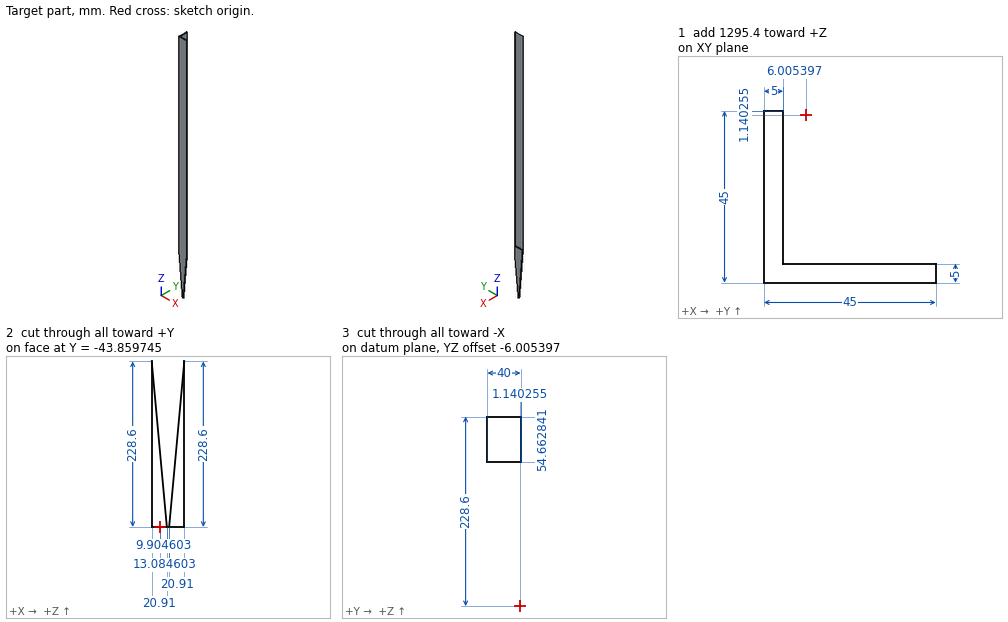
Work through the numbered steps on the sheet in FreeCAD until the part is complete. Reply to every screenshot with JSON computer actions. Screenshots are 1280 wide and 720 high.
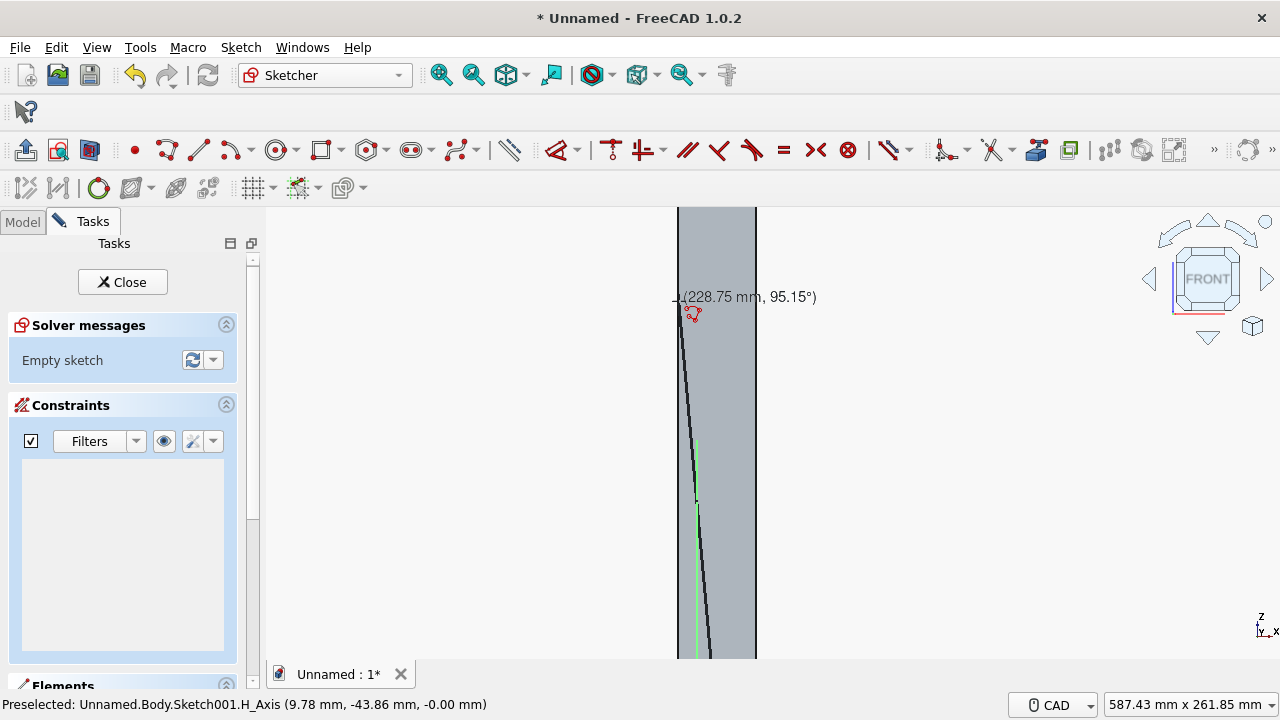
{"action": "left_click", "coordinate": [678, 301]}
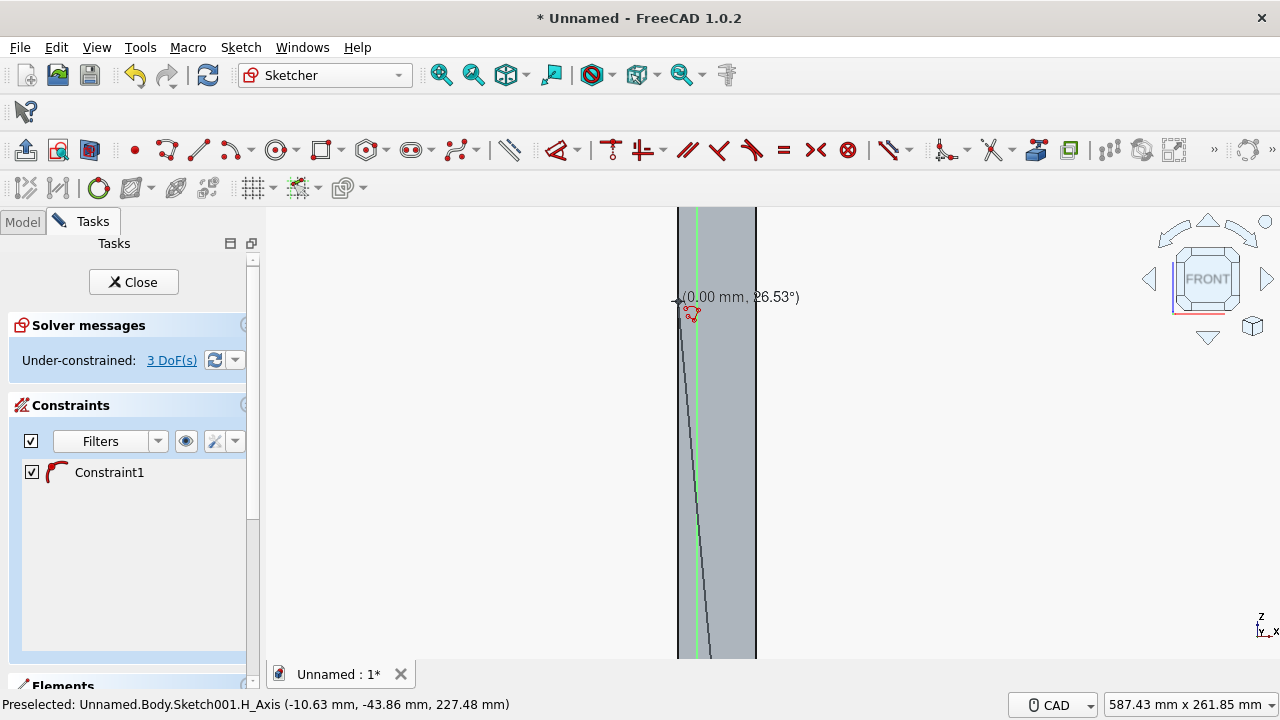
{"action": "scroll", "coordinate": [679, 300], "scroll_direction": "down", "scroll_amount": 2}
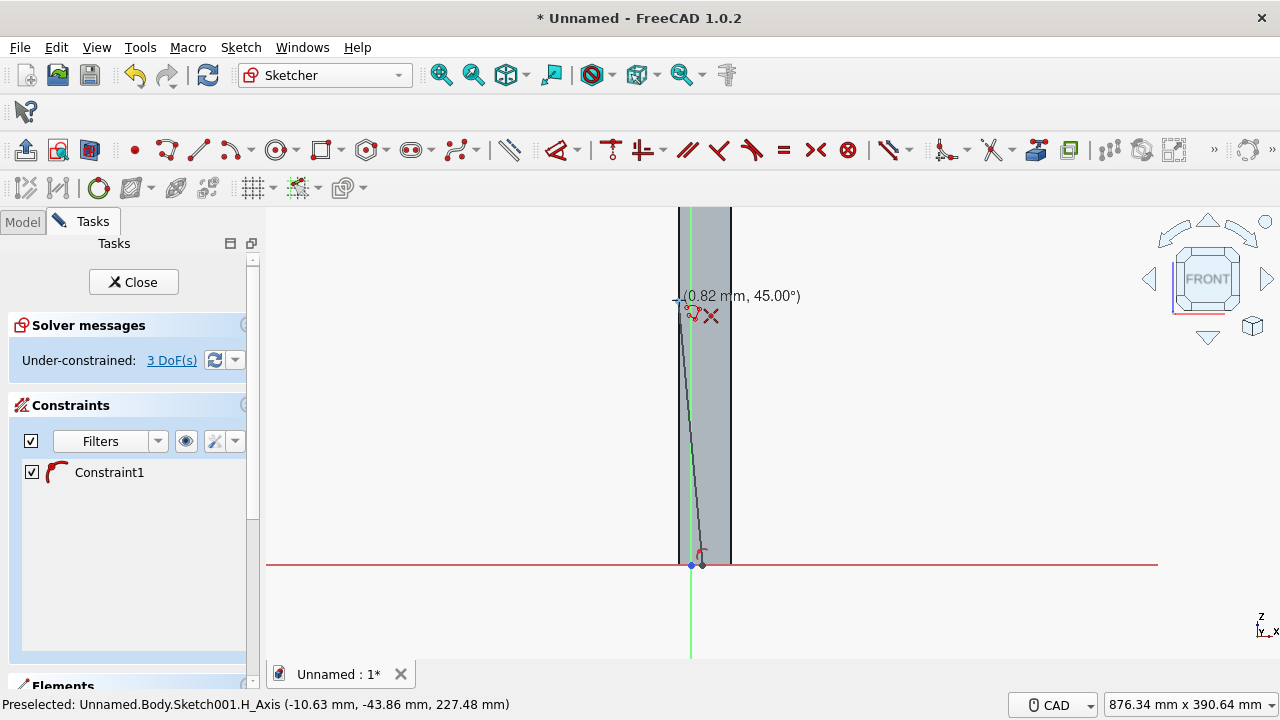
{"action": "scroll", "coordinate": [679, 565], "scroll_direction": "up", "scroll_amount": 2}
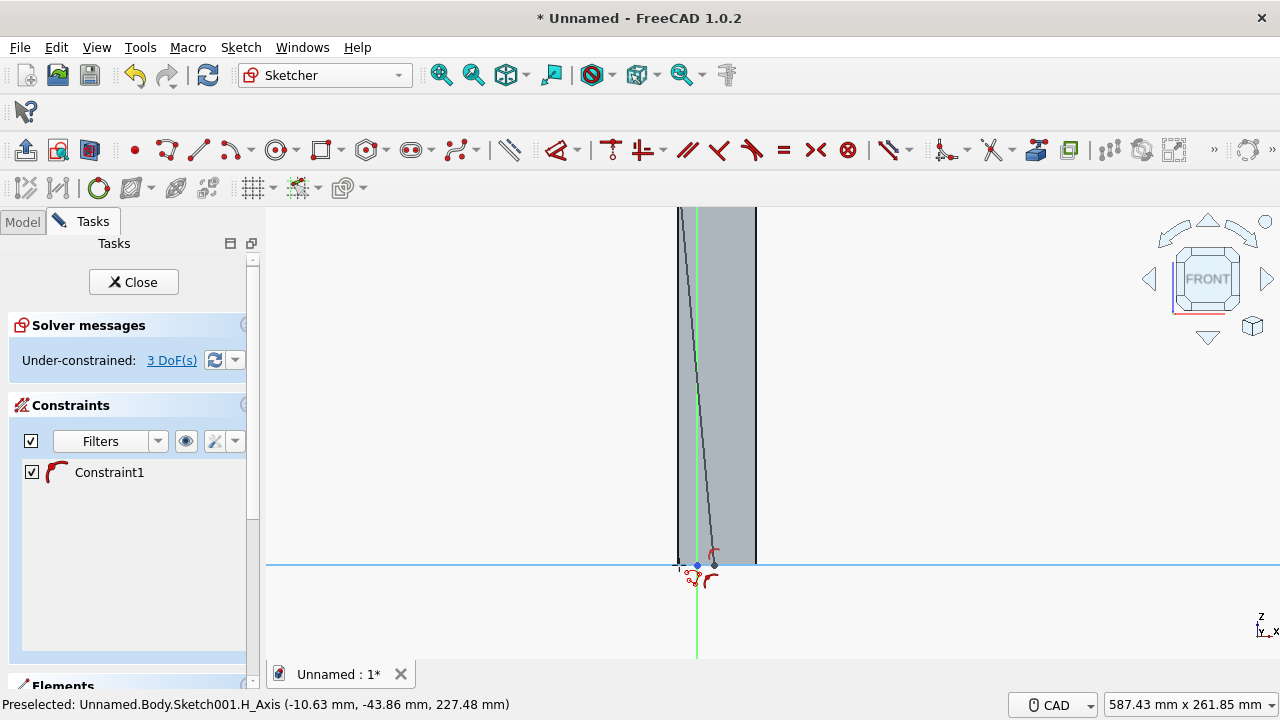
{"action": "left_click", "coordinate": [678, 556]}
{"action": "left_click", "coordinate": [714, 565]}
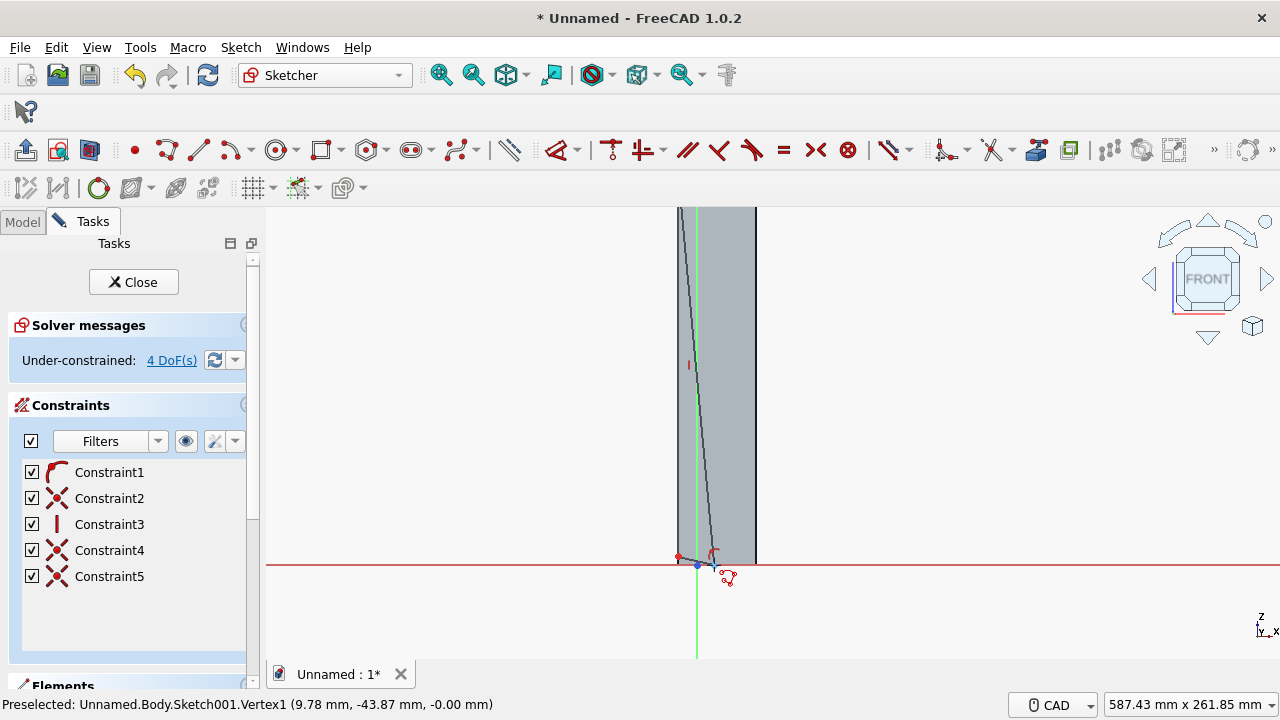
{"action": "scroll", "coordinate": [720, 565], "scroll_direction": "up", "scroll_amount": 6}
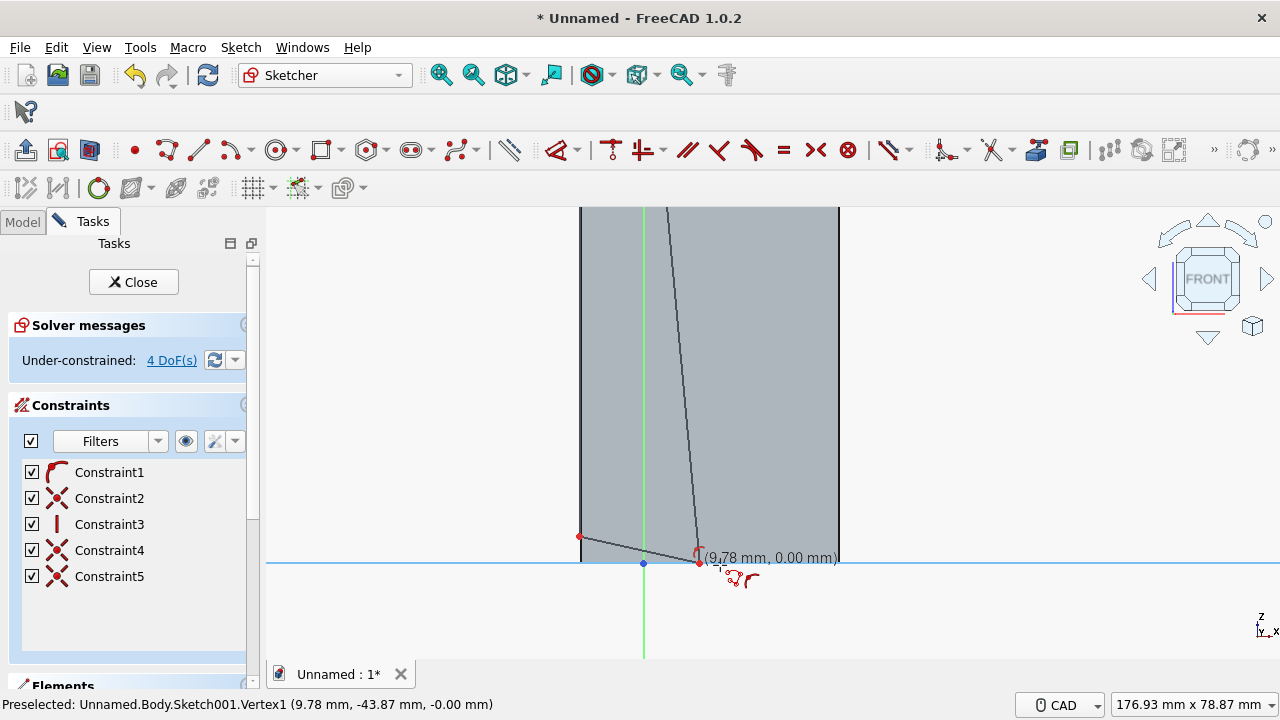
{"action": "left_click", "coordinate": [719, 563]}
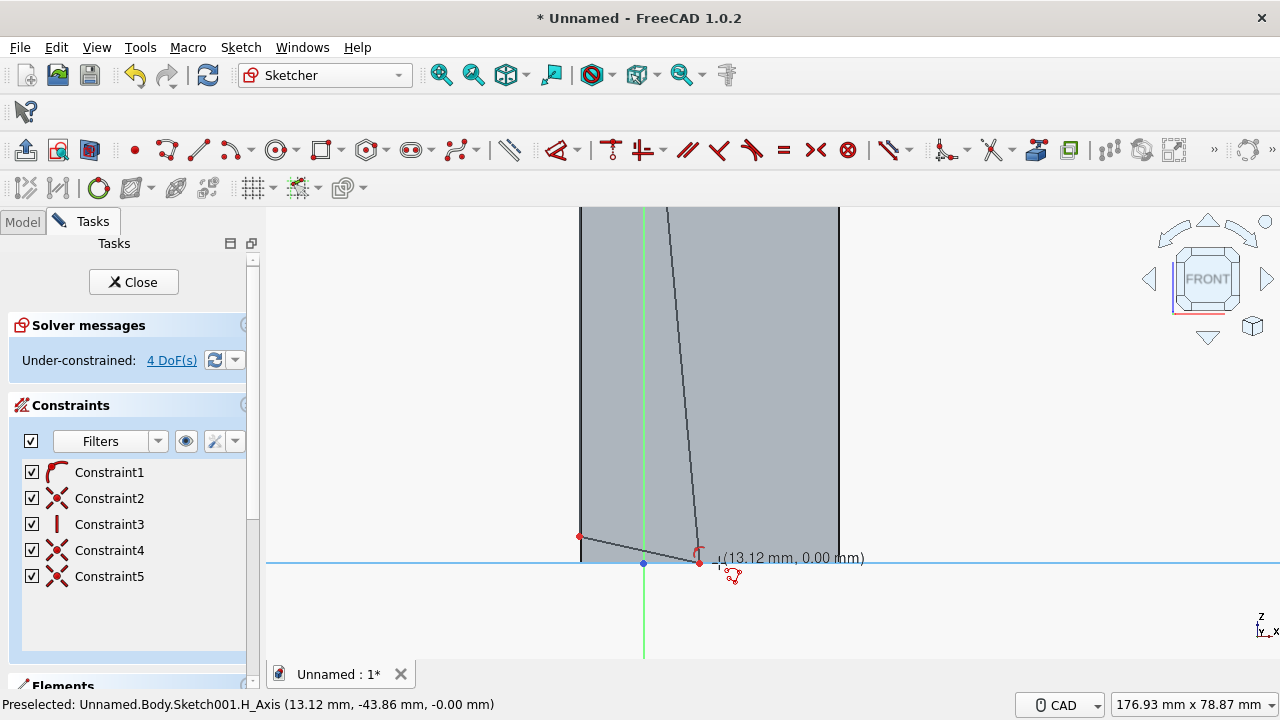
{"action": "scroll", "coordinate": [703, 566], "scroll_direction": "down", "scroll_amount": 8}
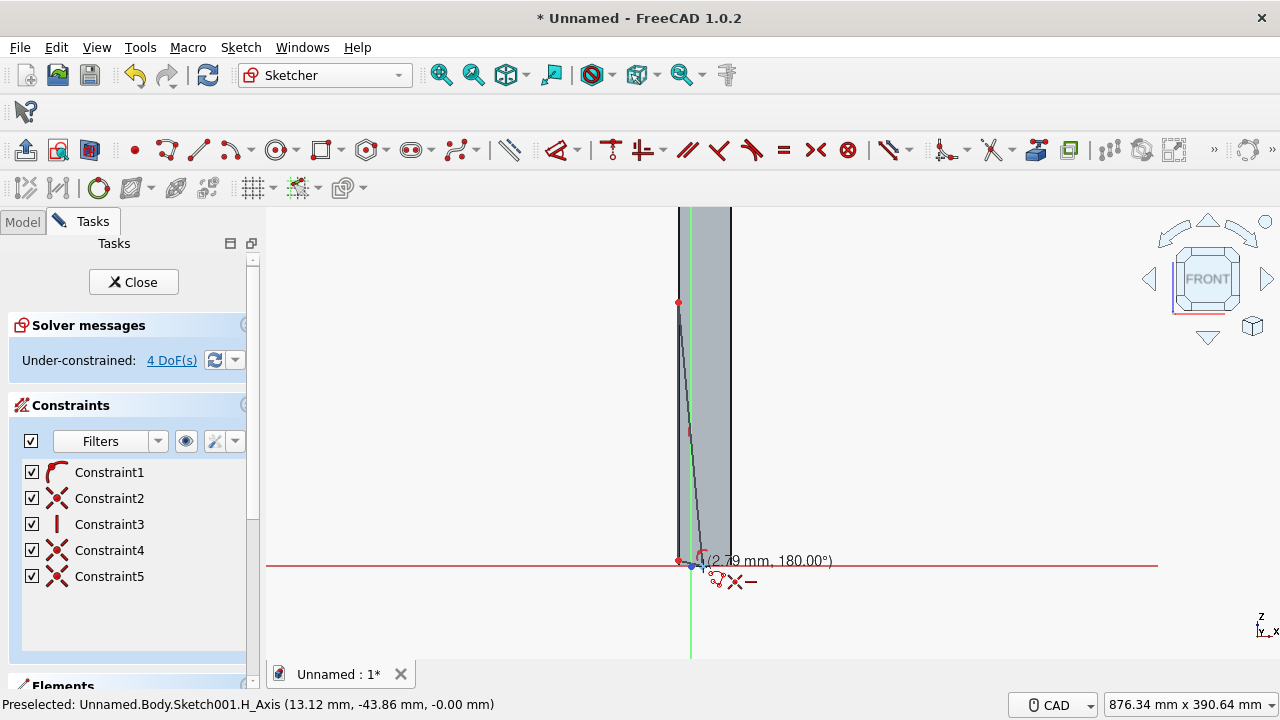
{"action": "left_click", "coordinate": [731, 557]}
{"action": "left_click", "coordinate": [731, 302]}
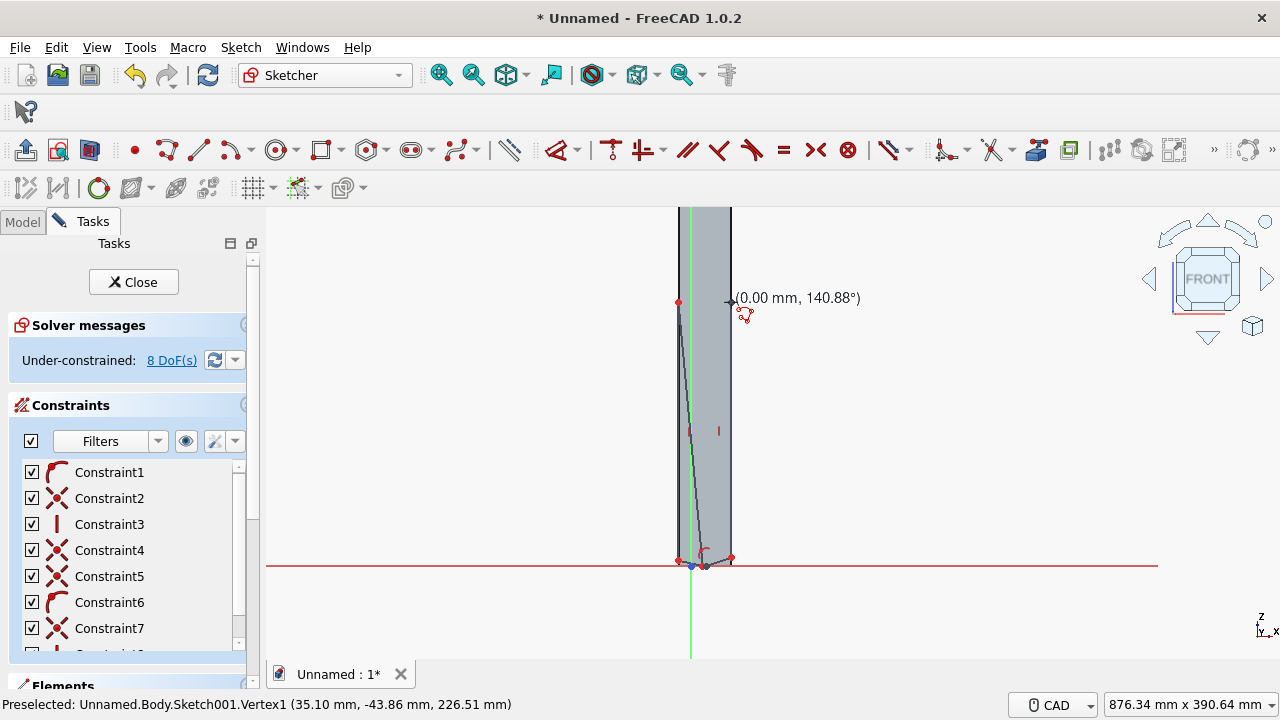
{"action": "scroll", "coordinate": [707, 566], "scroll_direction": "up", "scroll_amount": 8}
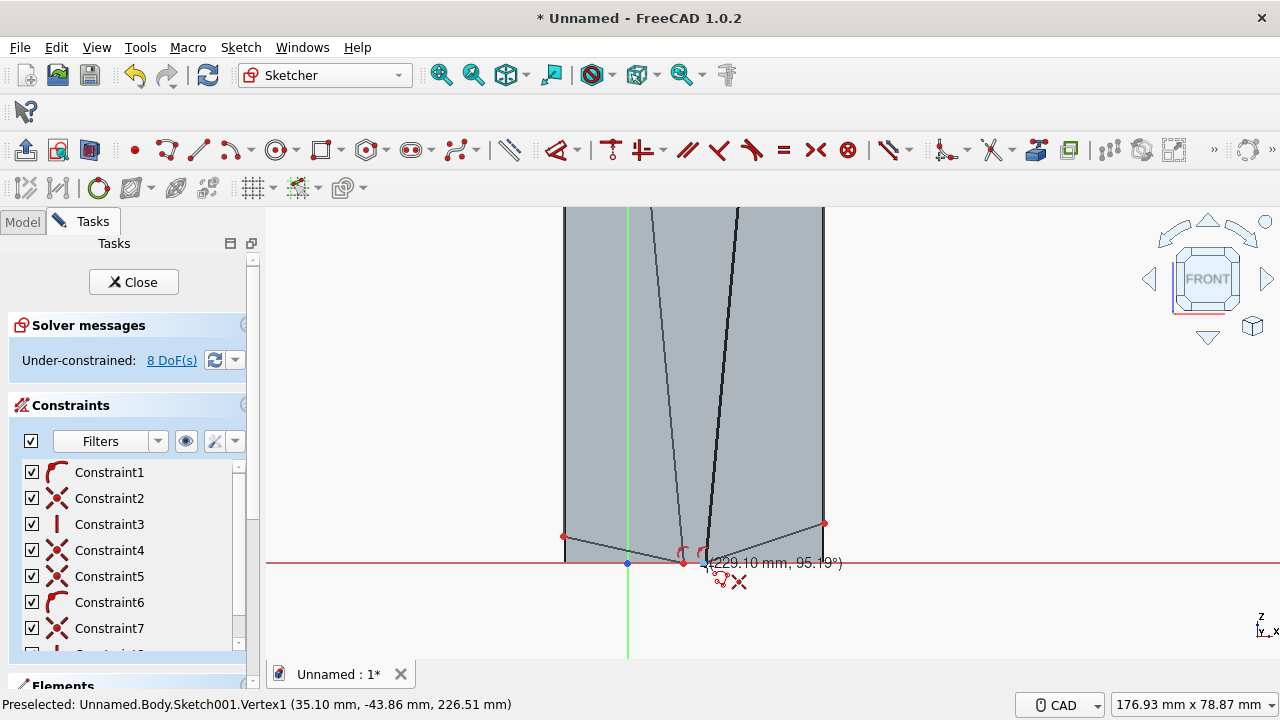
{"action": "left_click", "coordinate": [703, 563]}
{"action": "key", "text": "Escape"}
{"action": "key", "text": "Escape"}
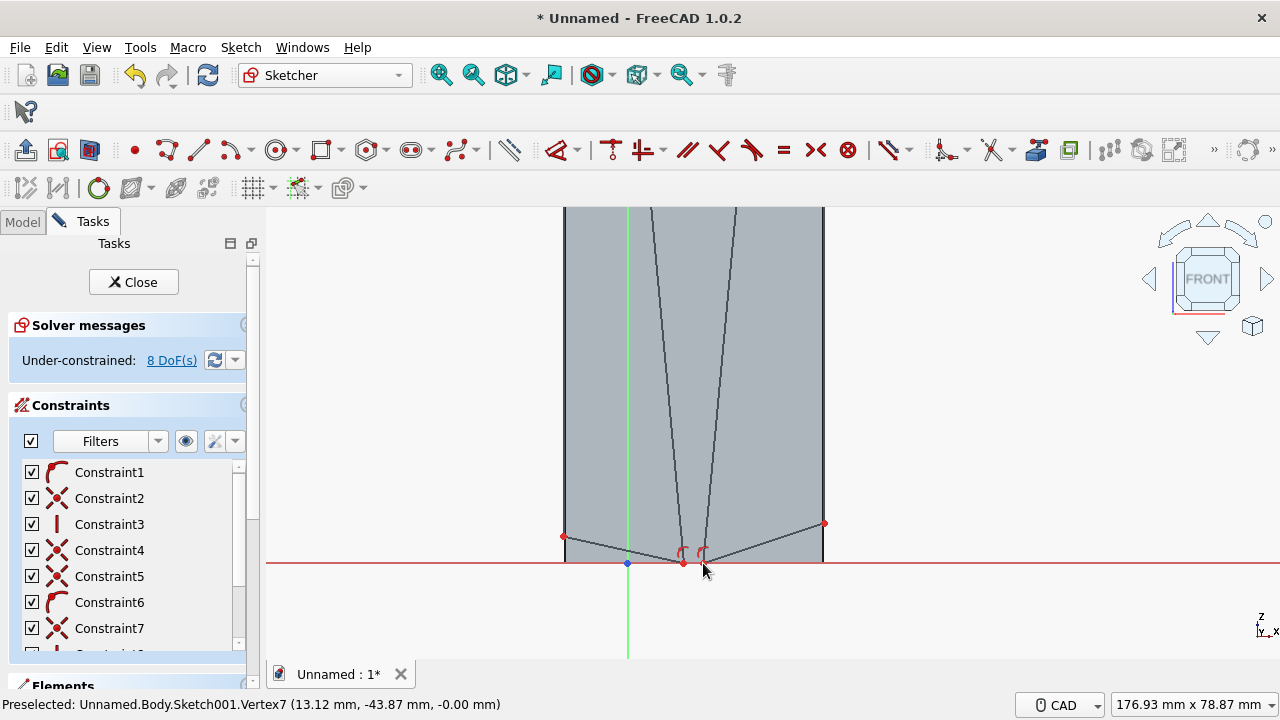
{"action": "left_click", "coordinate": [600, 545]}